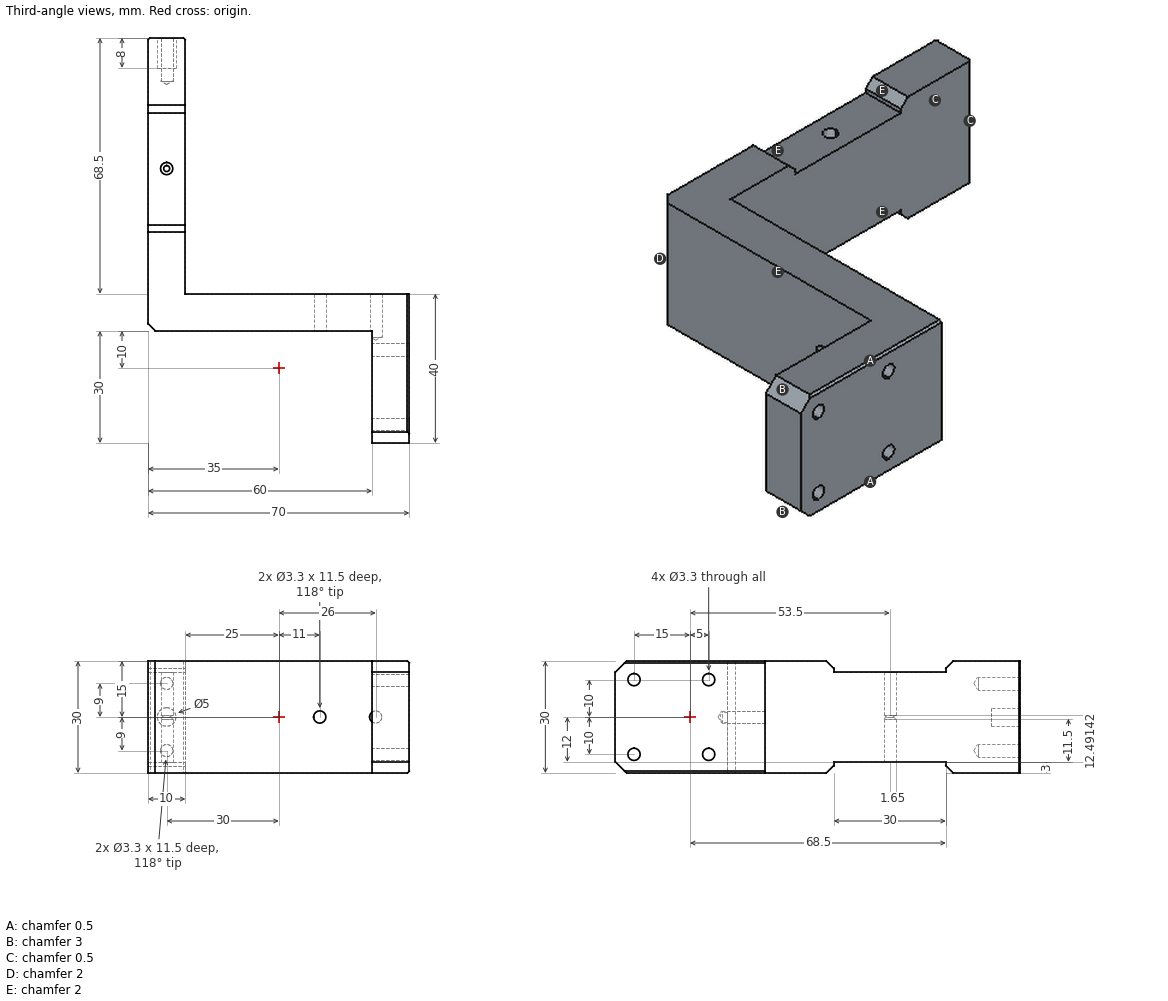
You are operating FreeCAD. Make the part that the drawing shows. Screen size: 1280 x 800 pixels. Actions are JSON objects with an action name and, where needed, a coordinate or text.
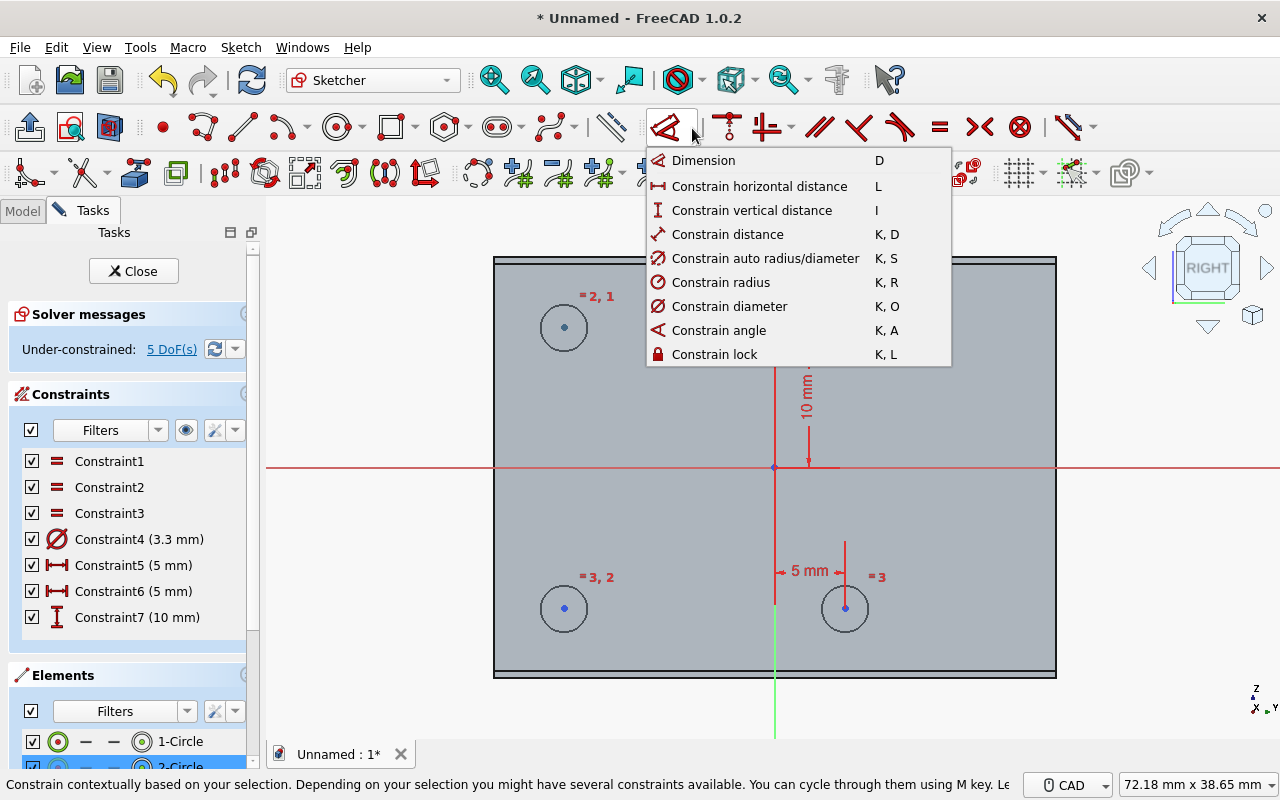
{"action": "left_click", "coordinate": [799, 186]}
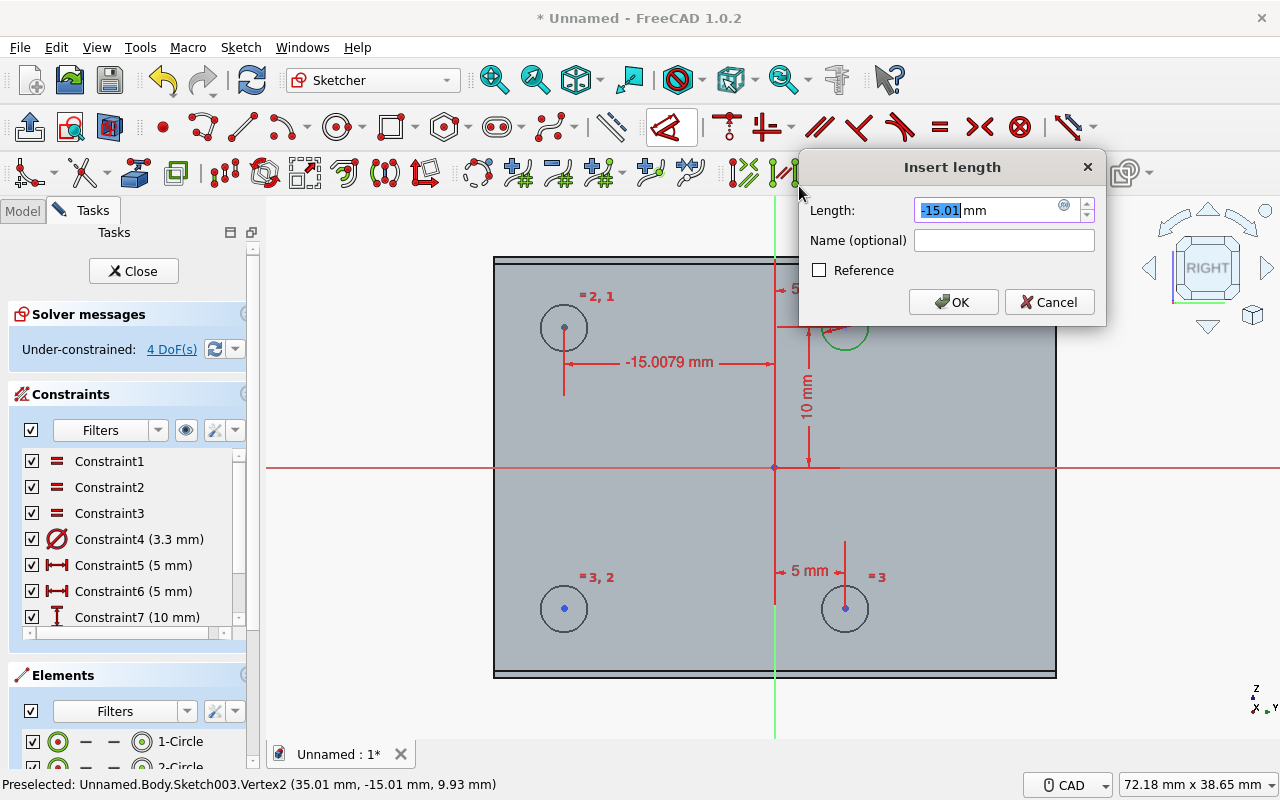
{"action": "type", "text": "-15"}
{"action": "key", "text": "Return"}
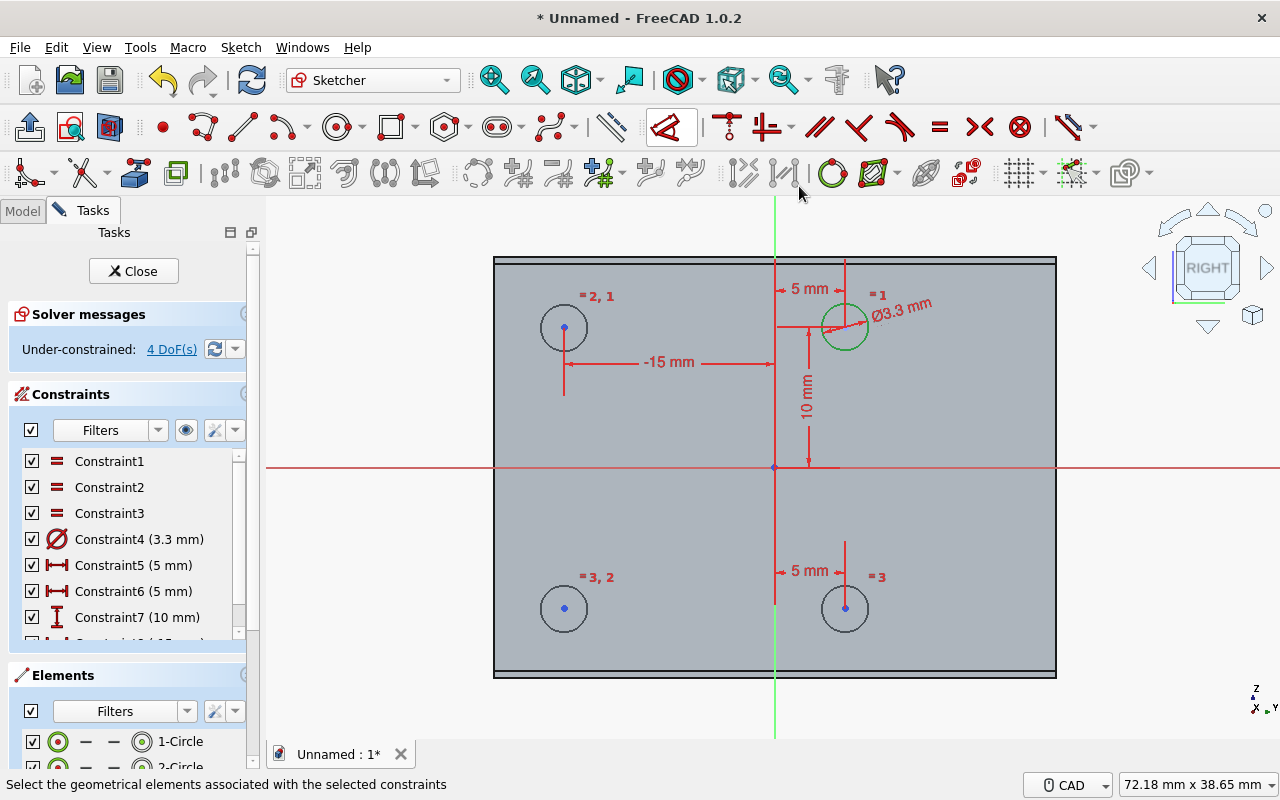
{"action": "left_click", "coordinate": [564, 328]}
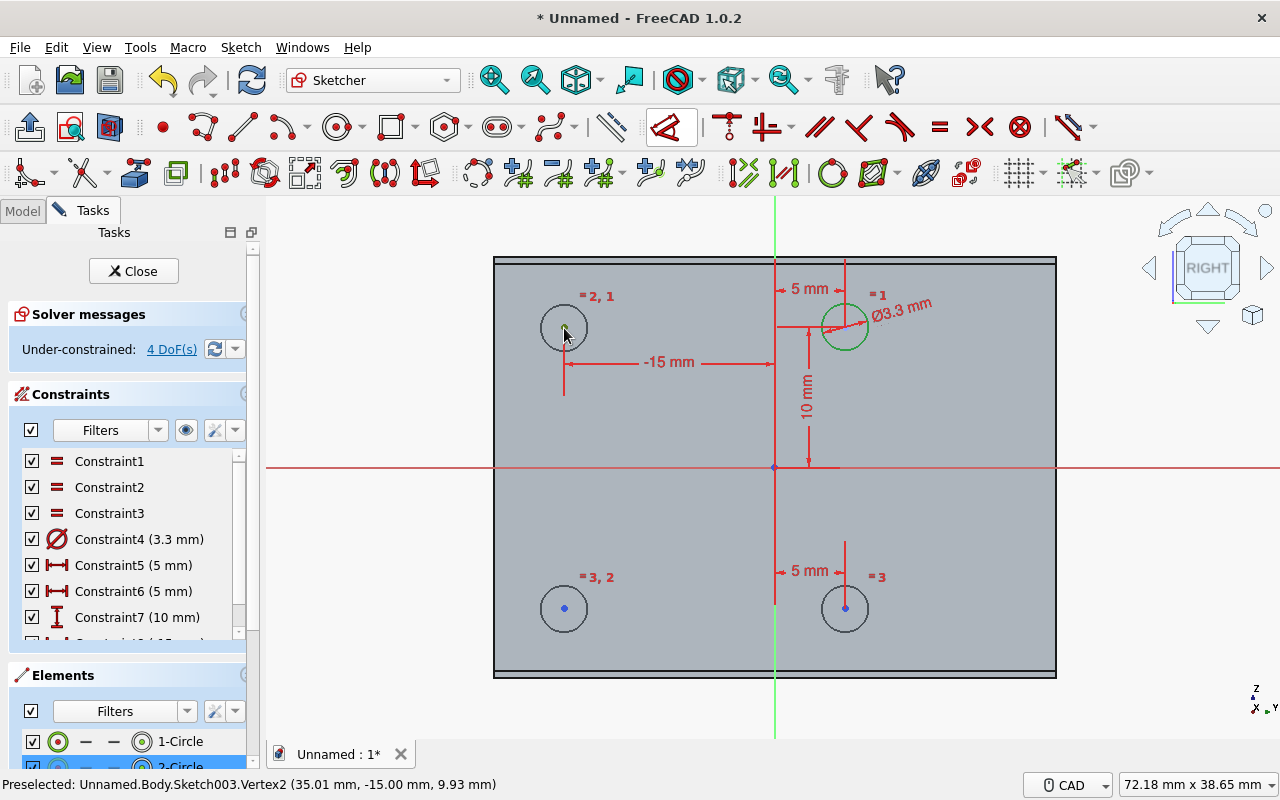
{"action": "left_click", "coordinate": [692, 128]}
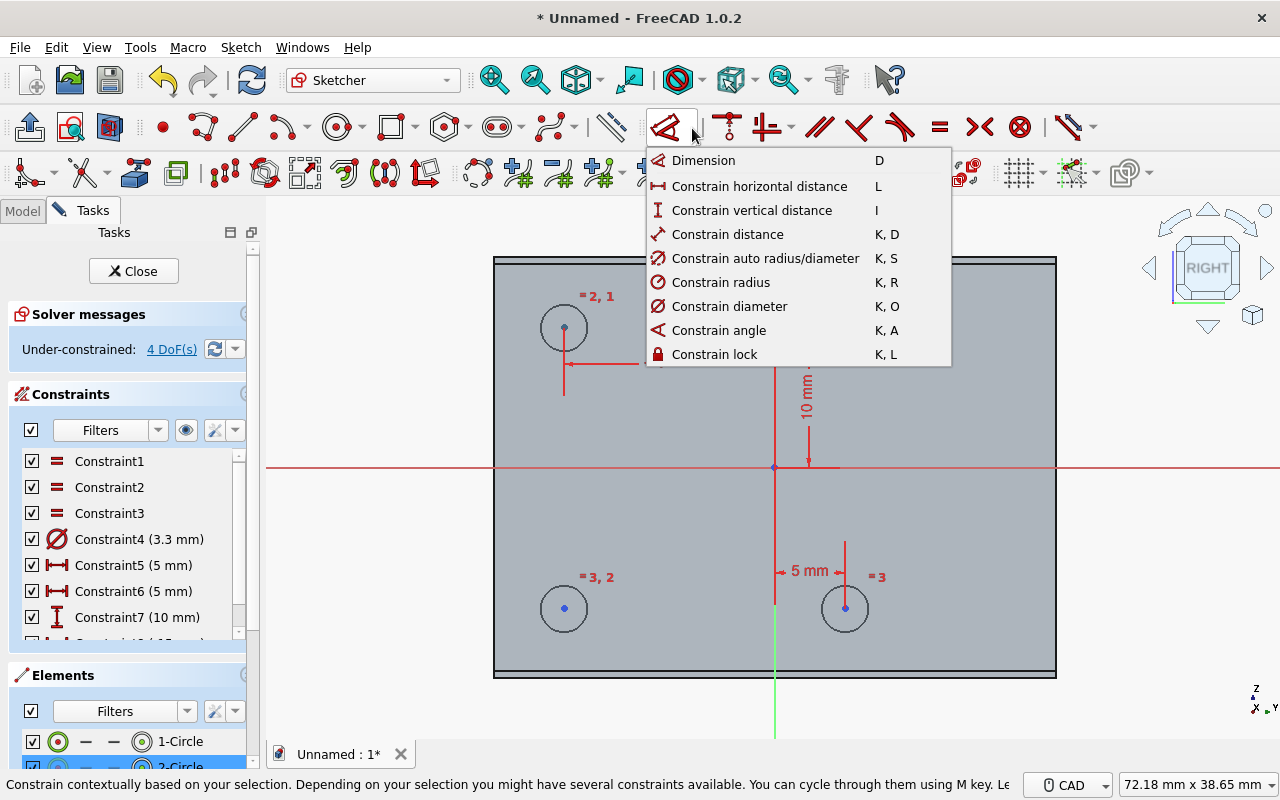
{"action": "left_click", "coordinate": [799, 210]}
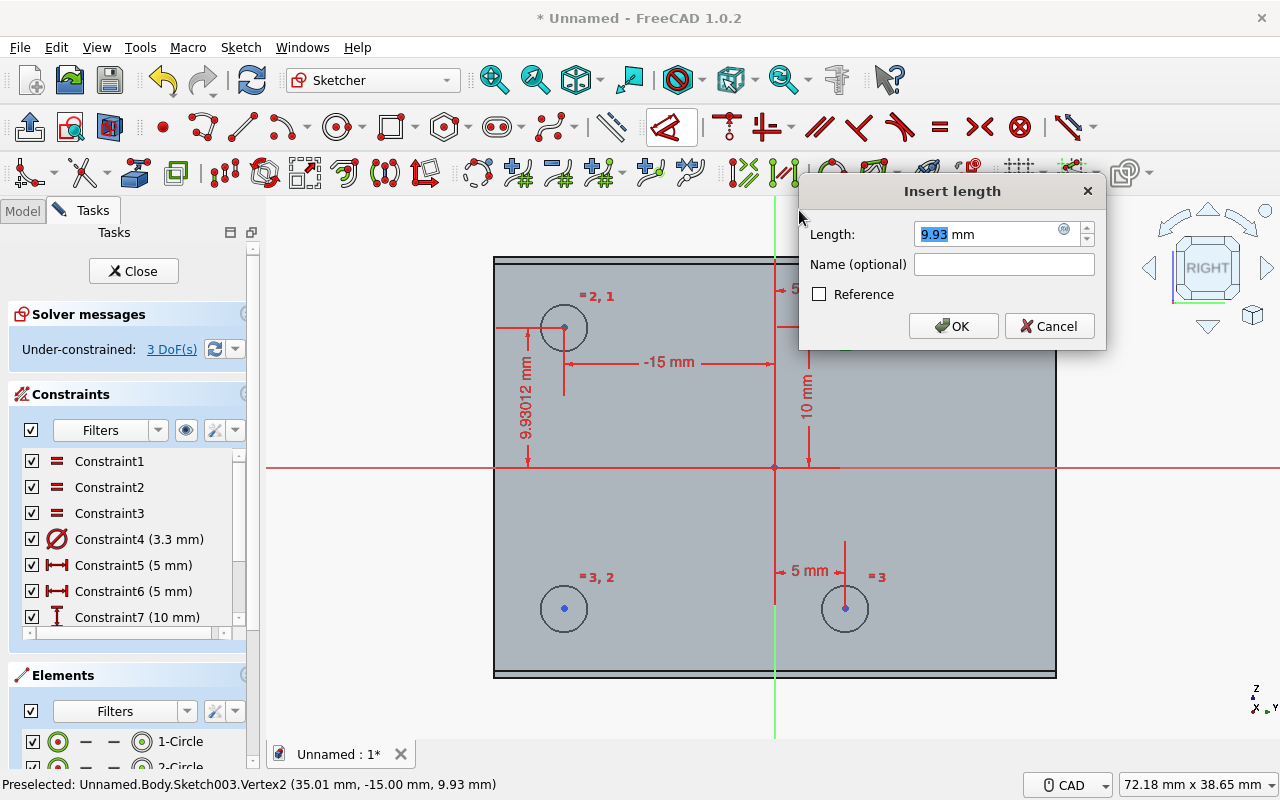
{"action": "type", "text": "10"}
{"action": "key", "text": "Return"}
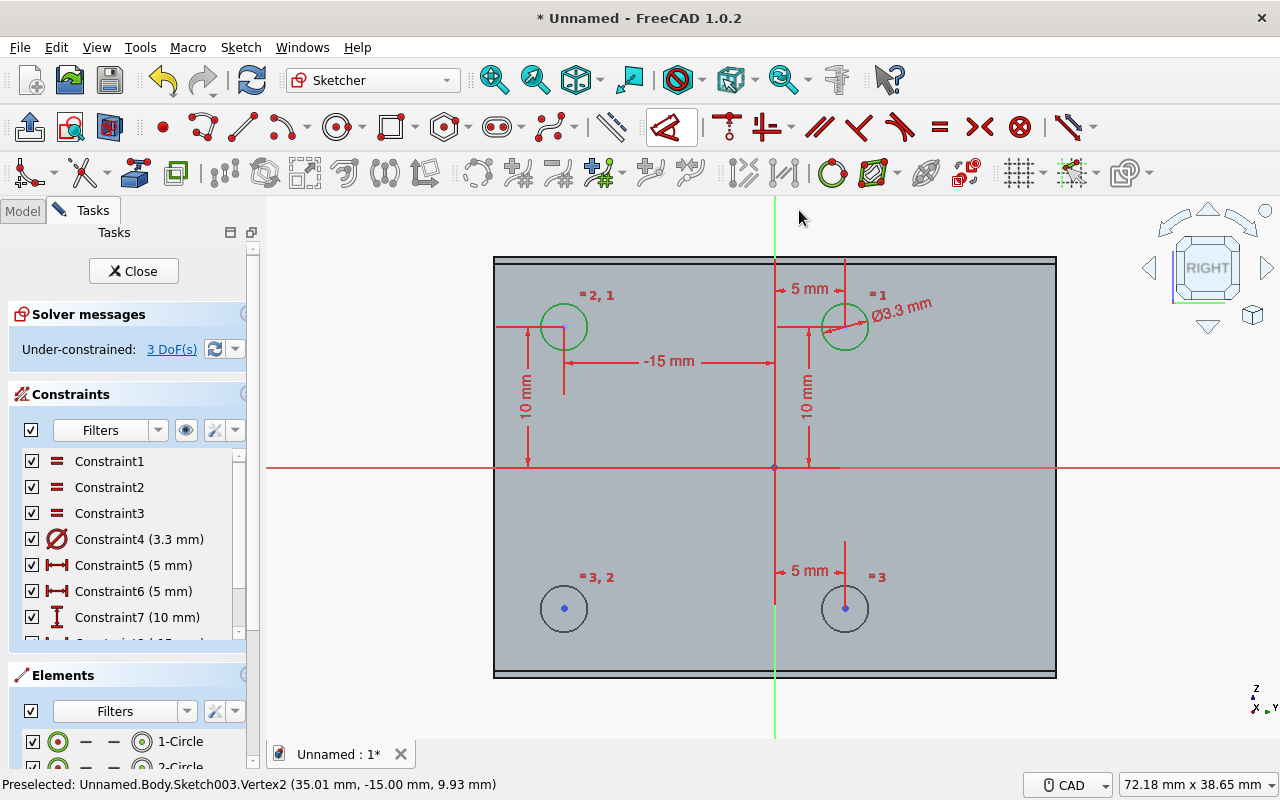
{"action": "left_click", "coordinate": [564, 609]}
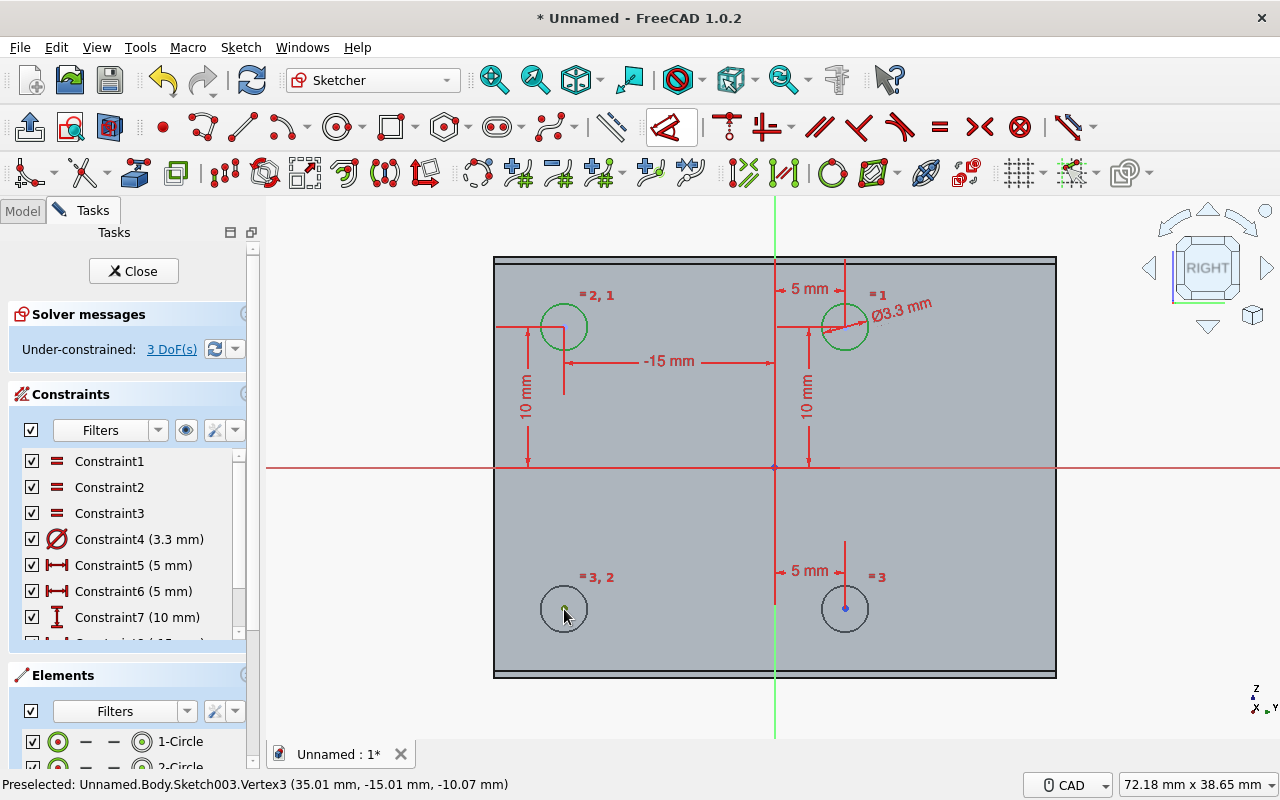
{"action": "key", "text": "l"}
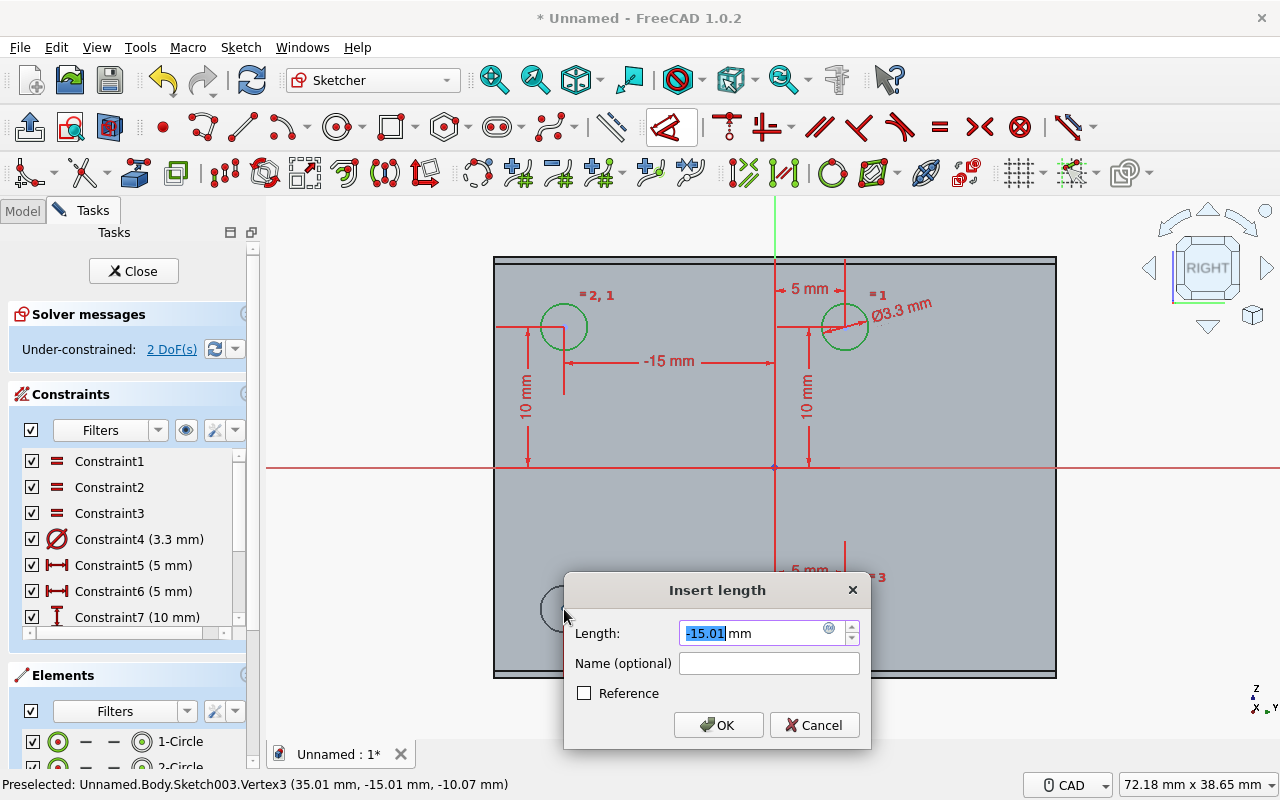
{"action": "type", "text": "-15"}
{"action": "key", "text": "Return"}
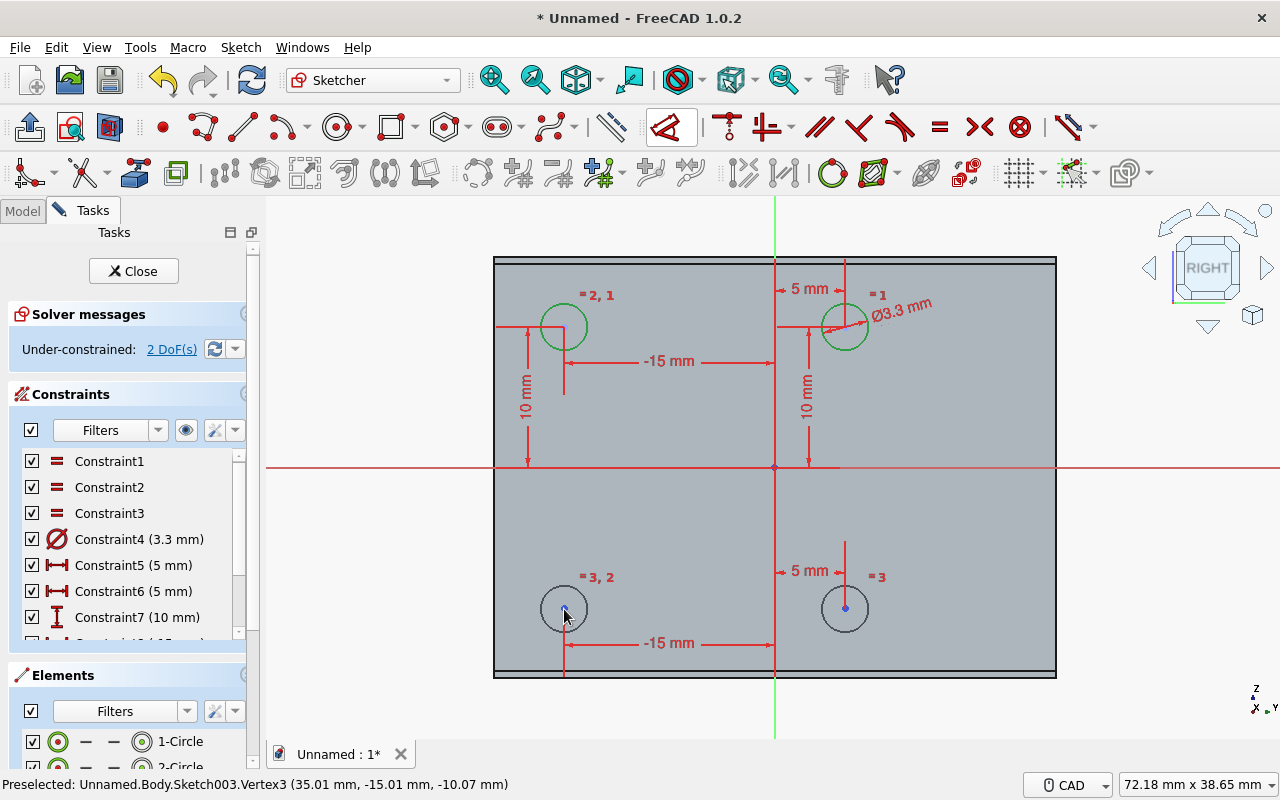
{"action": "left_click", "coordinate": [564, 609]}